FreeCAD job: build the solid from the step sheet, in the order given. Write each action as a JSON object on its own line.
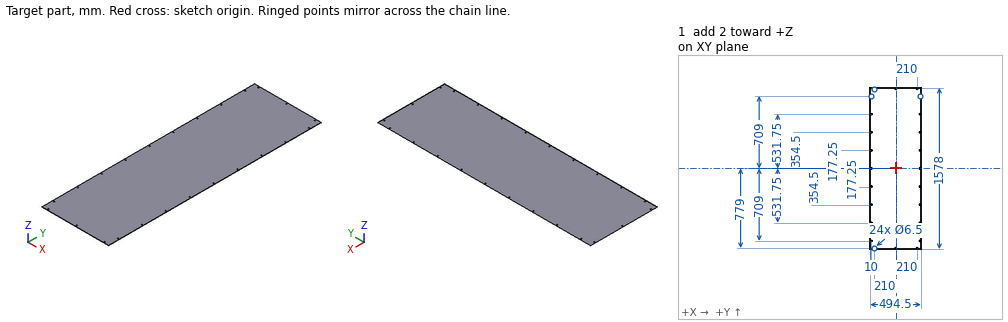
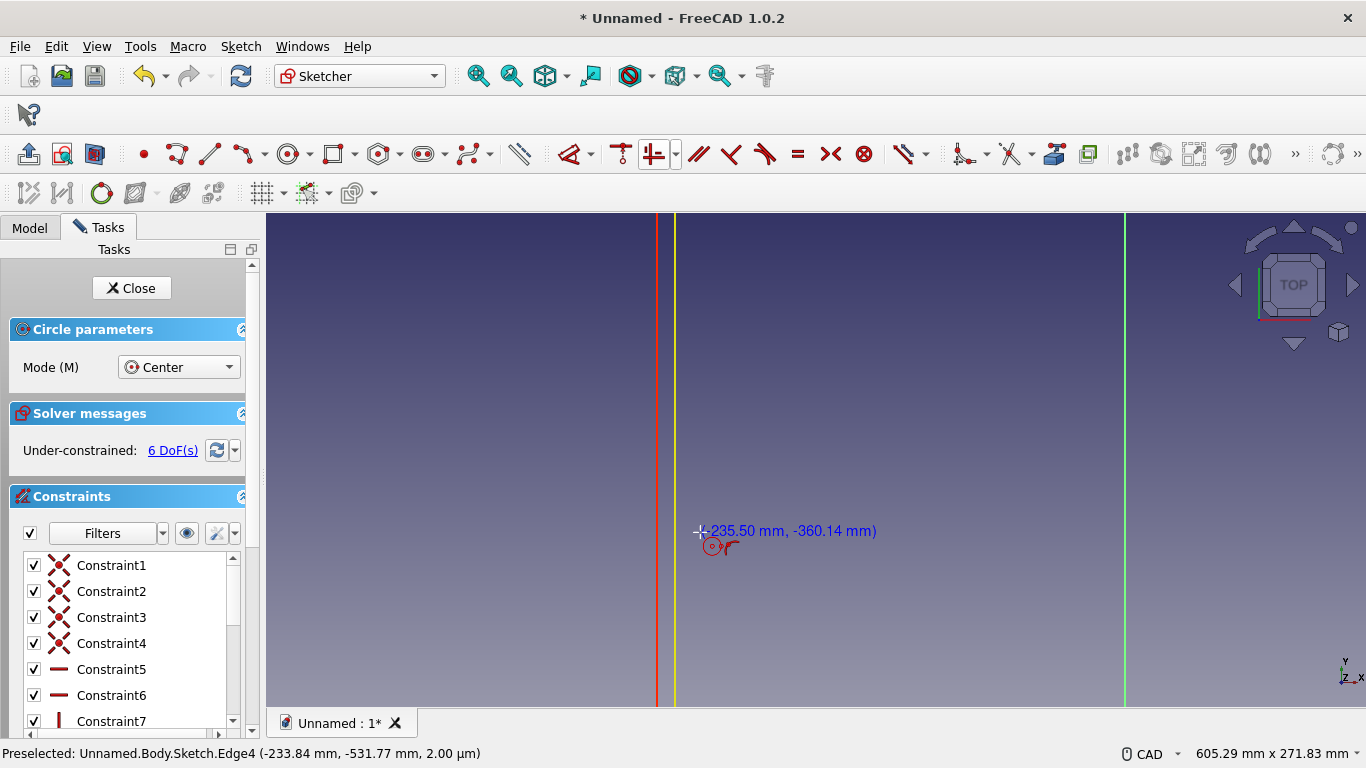
{"action": "left_click", "coordinate": [694, 526]}
{"action": "mouse_move", "coordinate": [698, 521]}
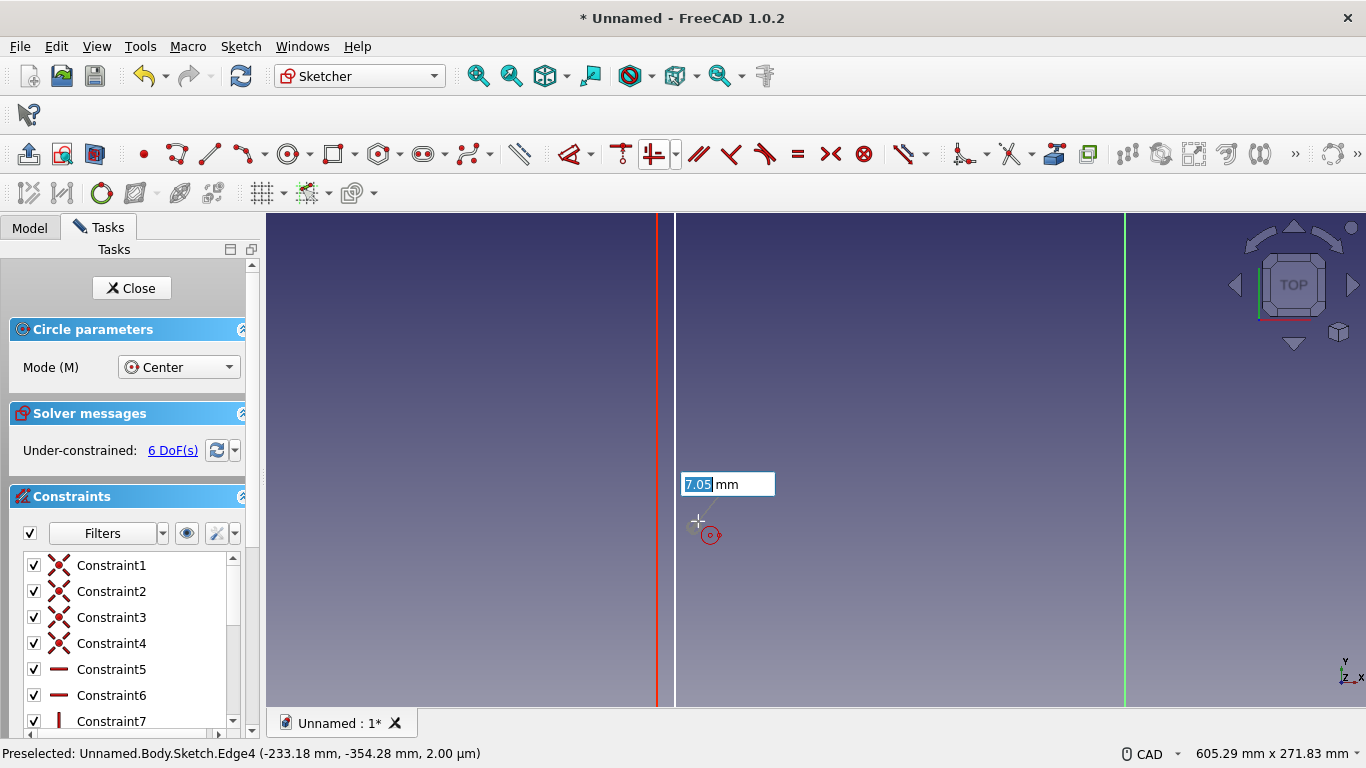
{"action": "type", "text": "6.5"}
{"action": "key", "text": "Return"}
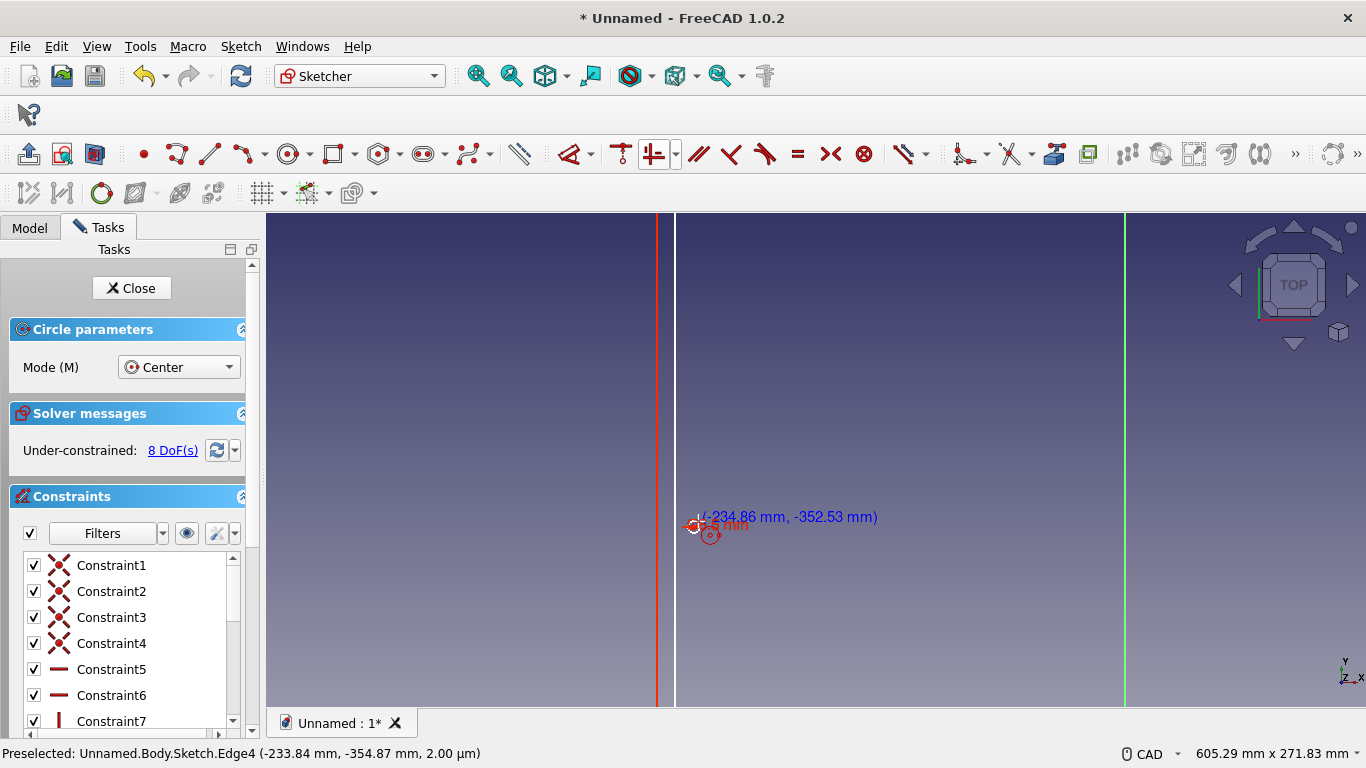
{"action": "scroll", "coordinate": [700, 532], "scroll_direction": "down", "scroll_amount": 11}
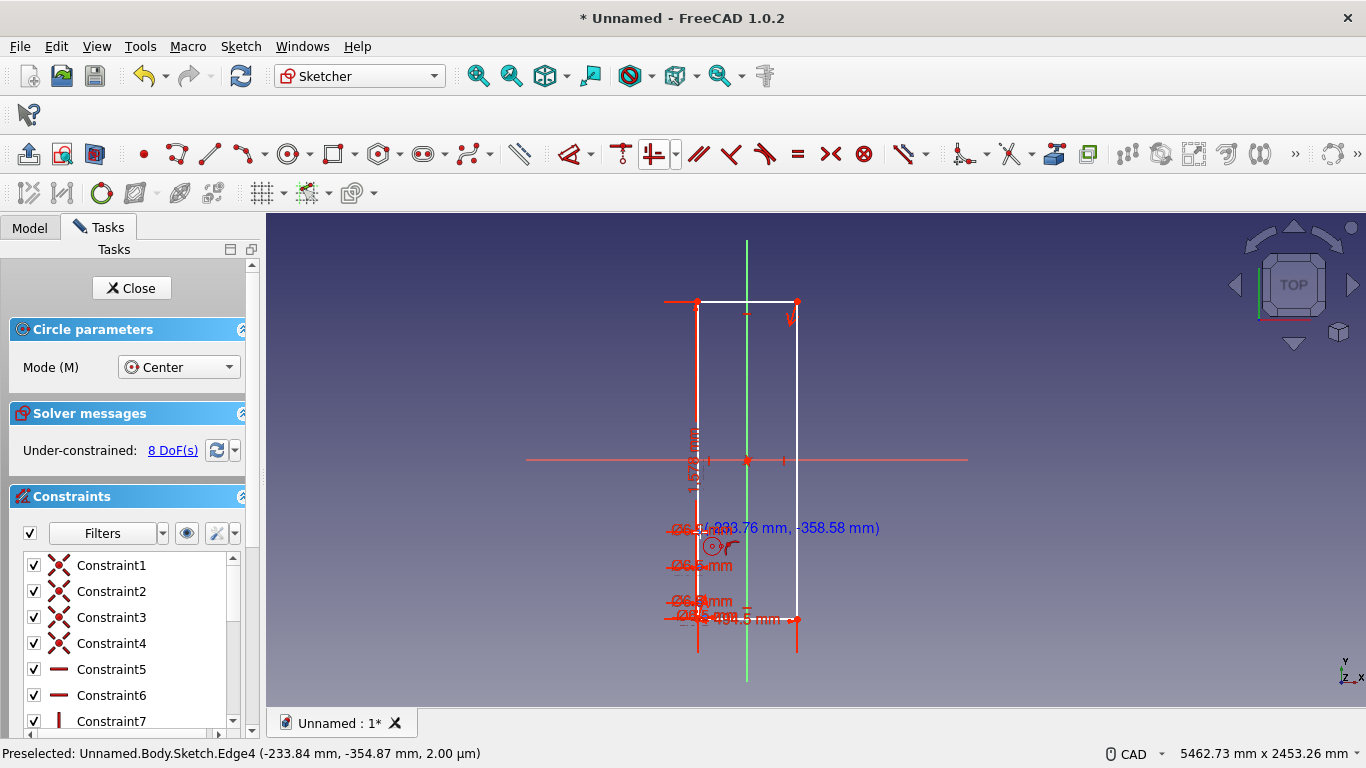
{"action": "scroll", "coordinate": [700, 496], "scroll_direction": "up", "scroll_amount": 18}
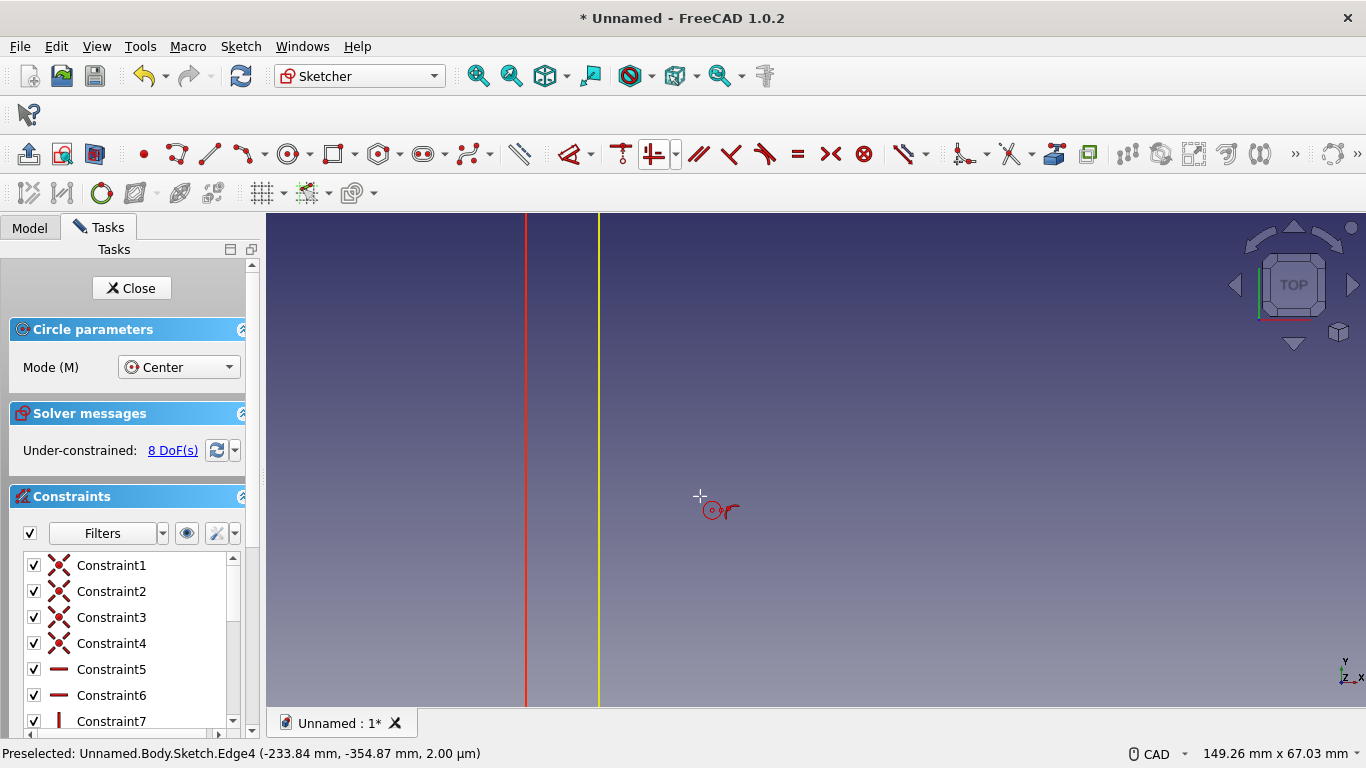
{"action": "scroll", "coordinate": [700, 496], "scroll_direction": "down", "scroll_amount": 18}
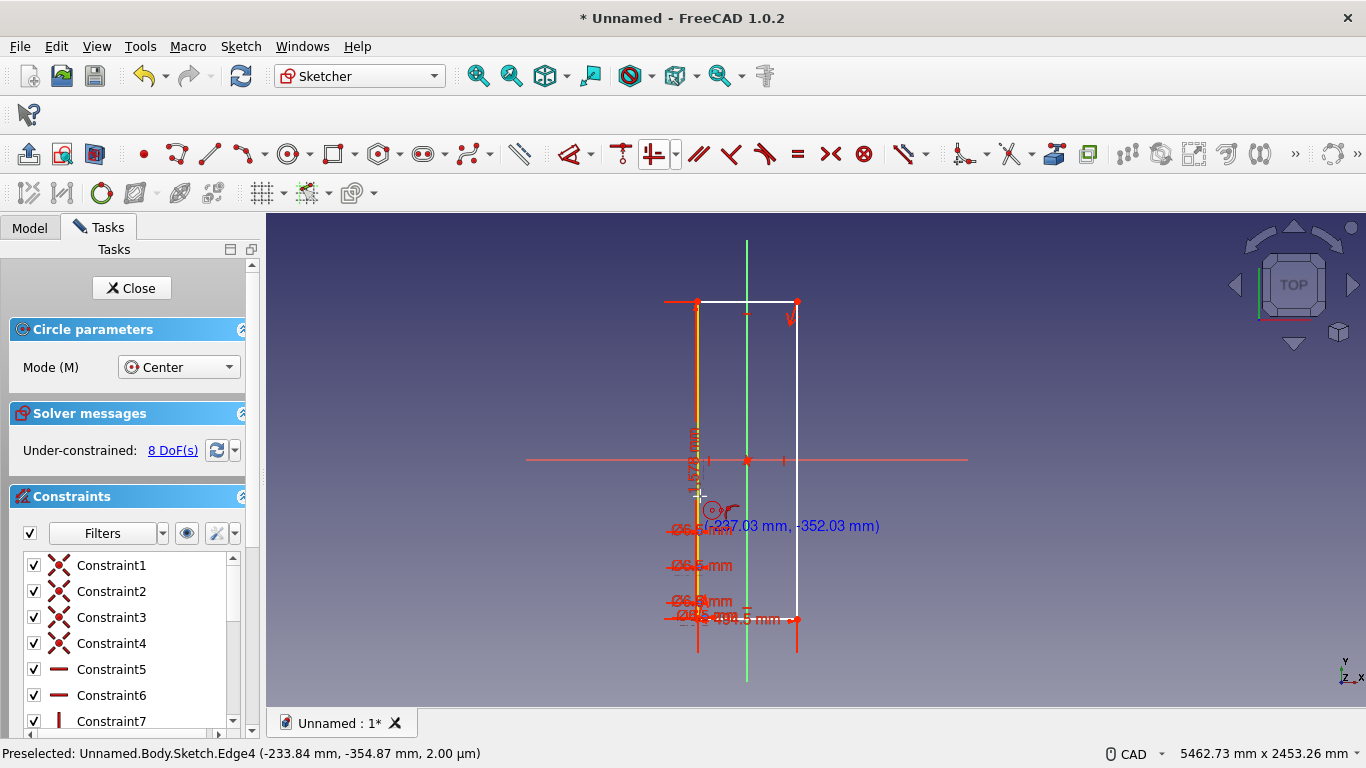
{"action": "scroll", "coordinate": [700, 496], "scroll_direction": "up", "scroll_amount": 11}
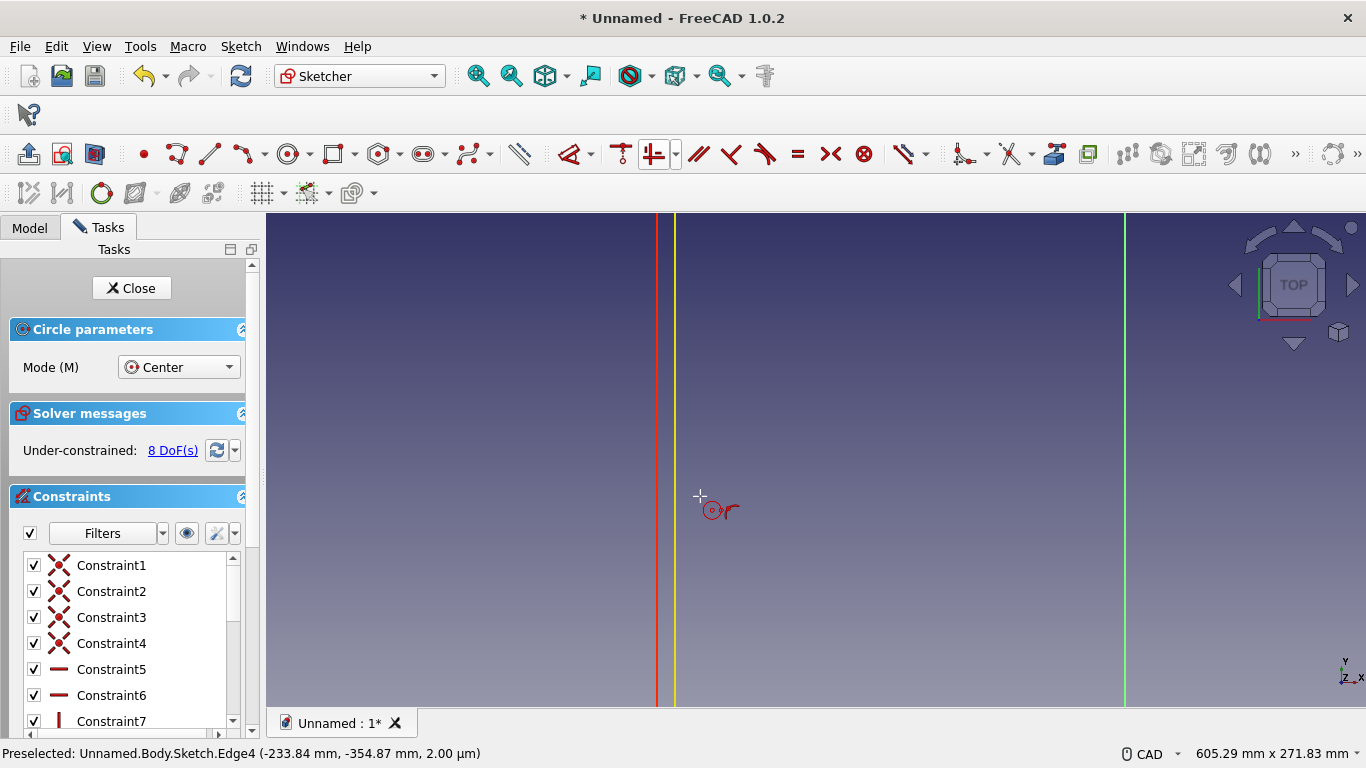
{"action": "left_click", "coordinate": [694, 493]}
{"action": "mouse_move", "coordinate": [698, 489]}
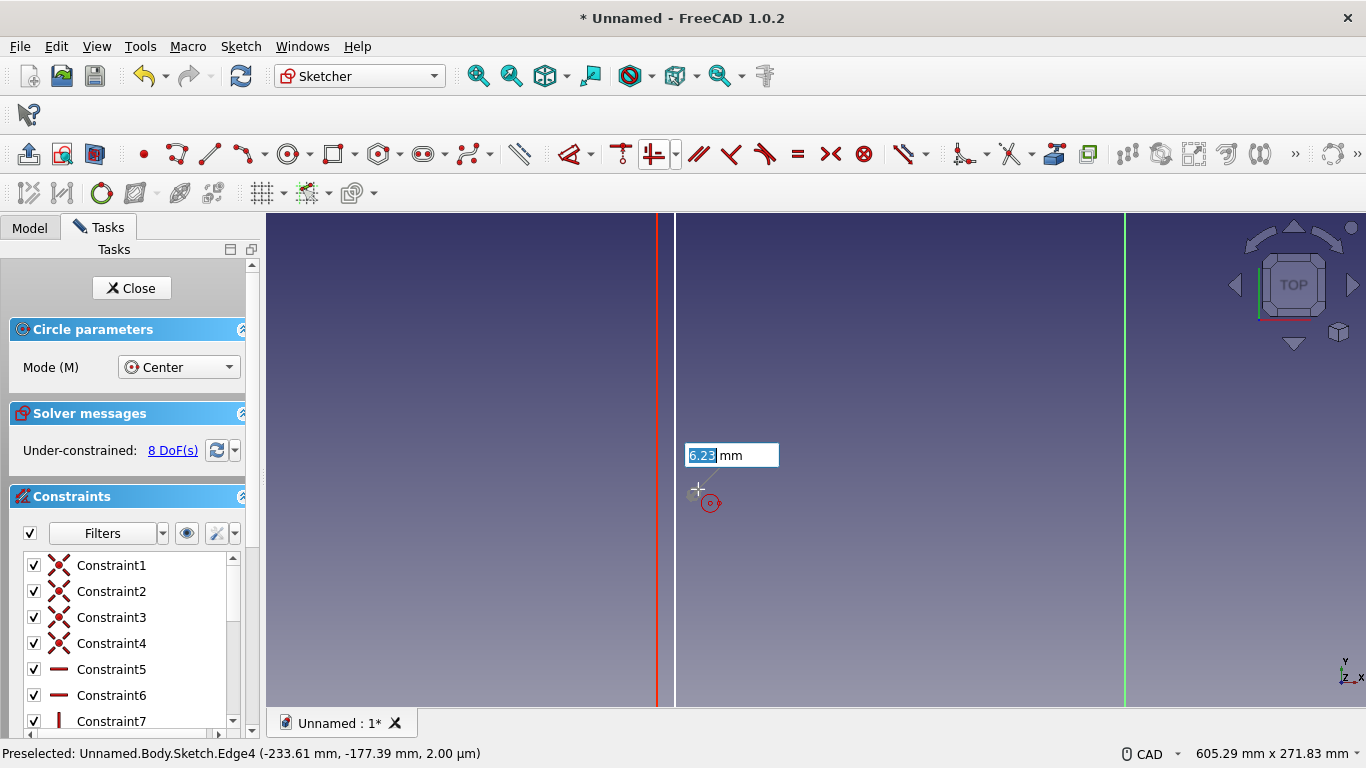
{"action": "type", "text": "6.5"}
{"action": "key", "text": "Return"}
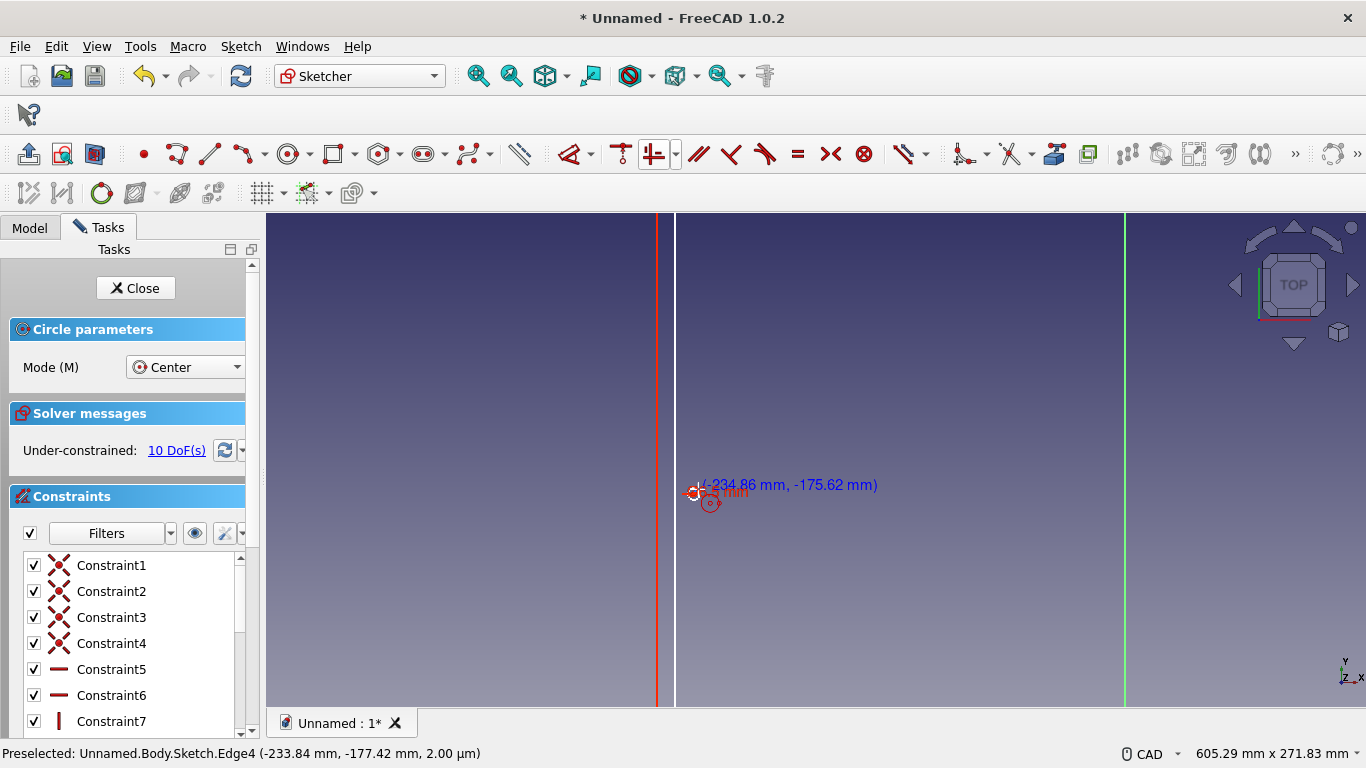
{"action": "scroll", "coordinate": [700, 496], "scroll_direction": "down", "scroll_amount": 11}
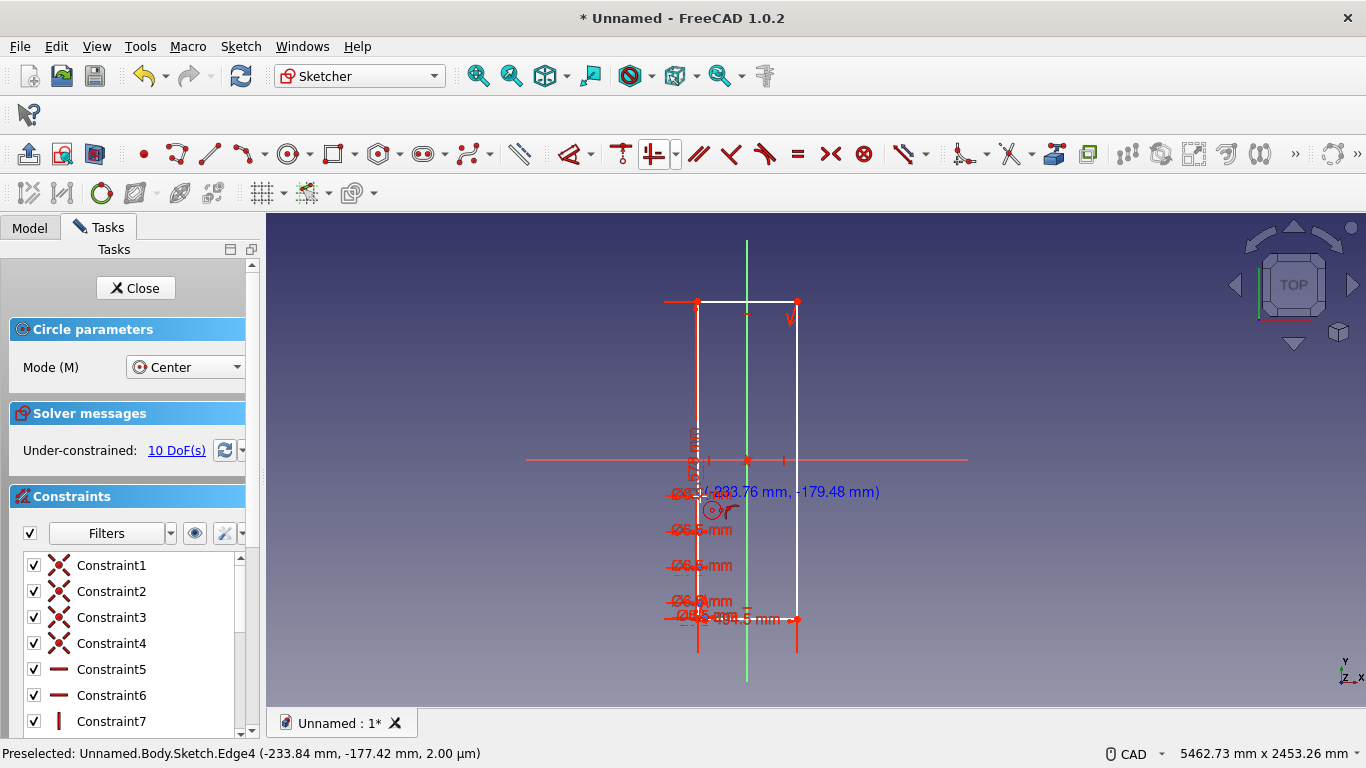
{"action": "scroll", "coordinate": [747, 617], "scroll_direction": "up", "scroll_amount": 18}